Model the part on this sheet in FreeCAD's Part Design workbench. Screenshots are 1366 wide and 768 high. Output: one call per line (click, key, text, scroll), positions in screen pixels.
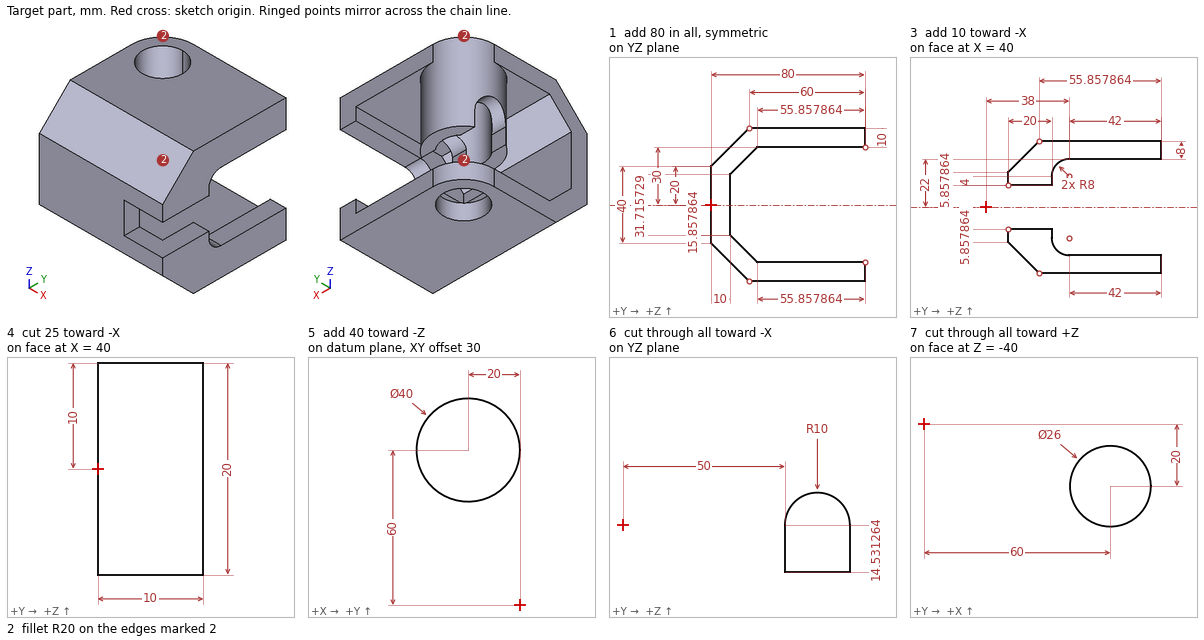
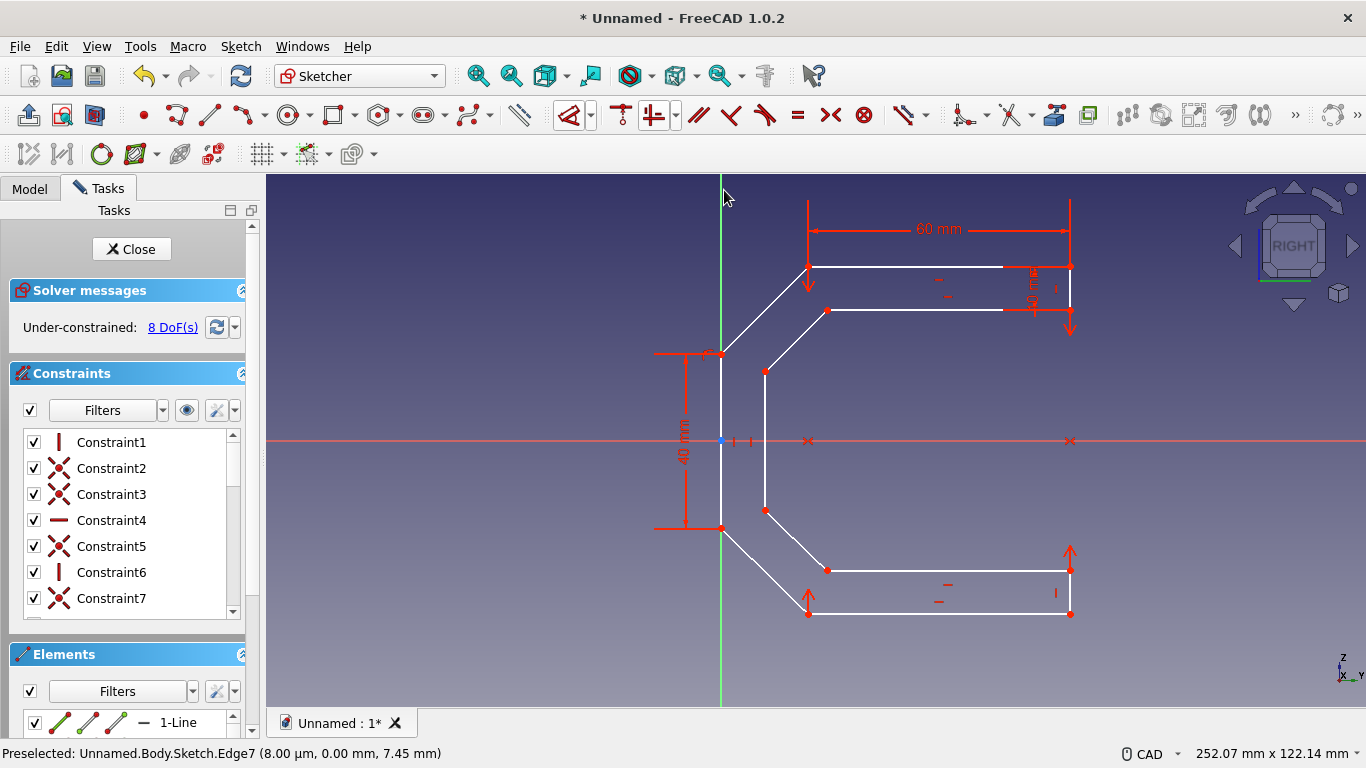
click(765, 511)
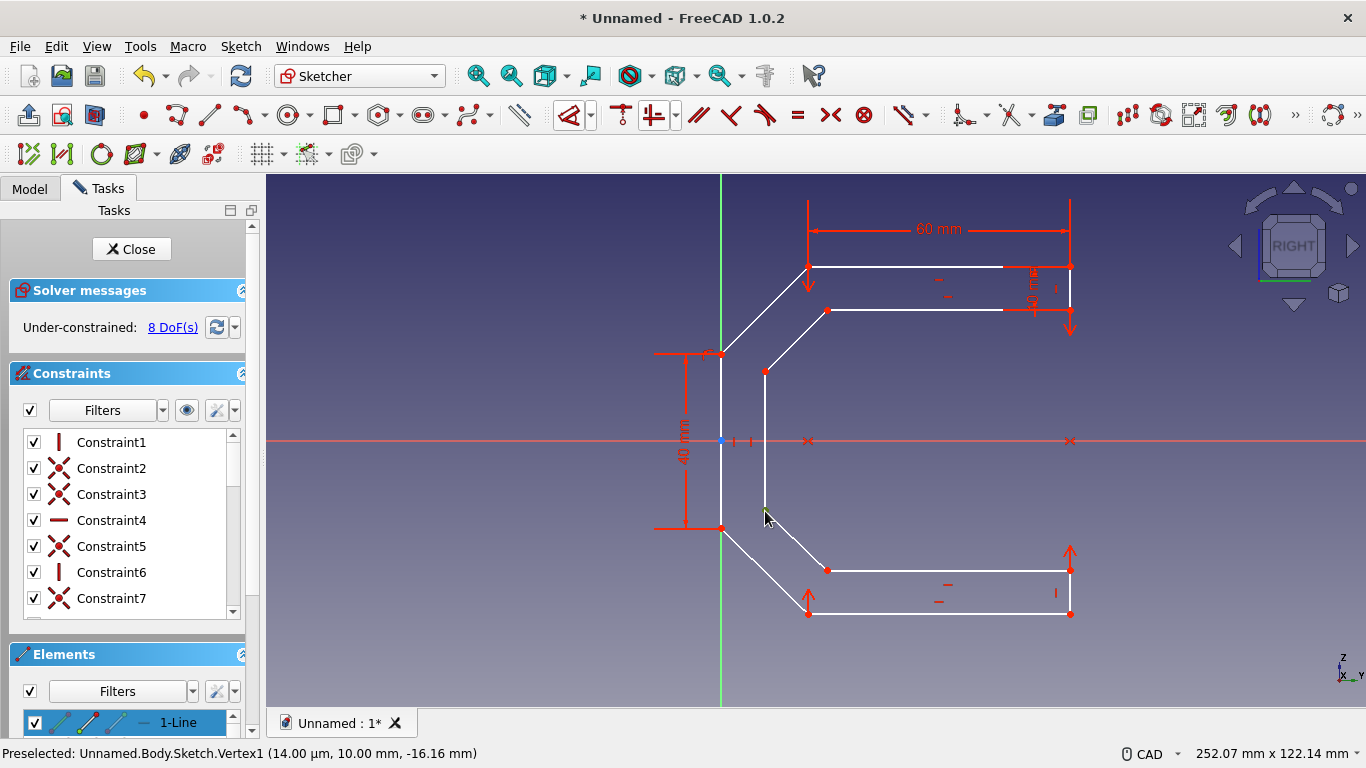
click(590, 116)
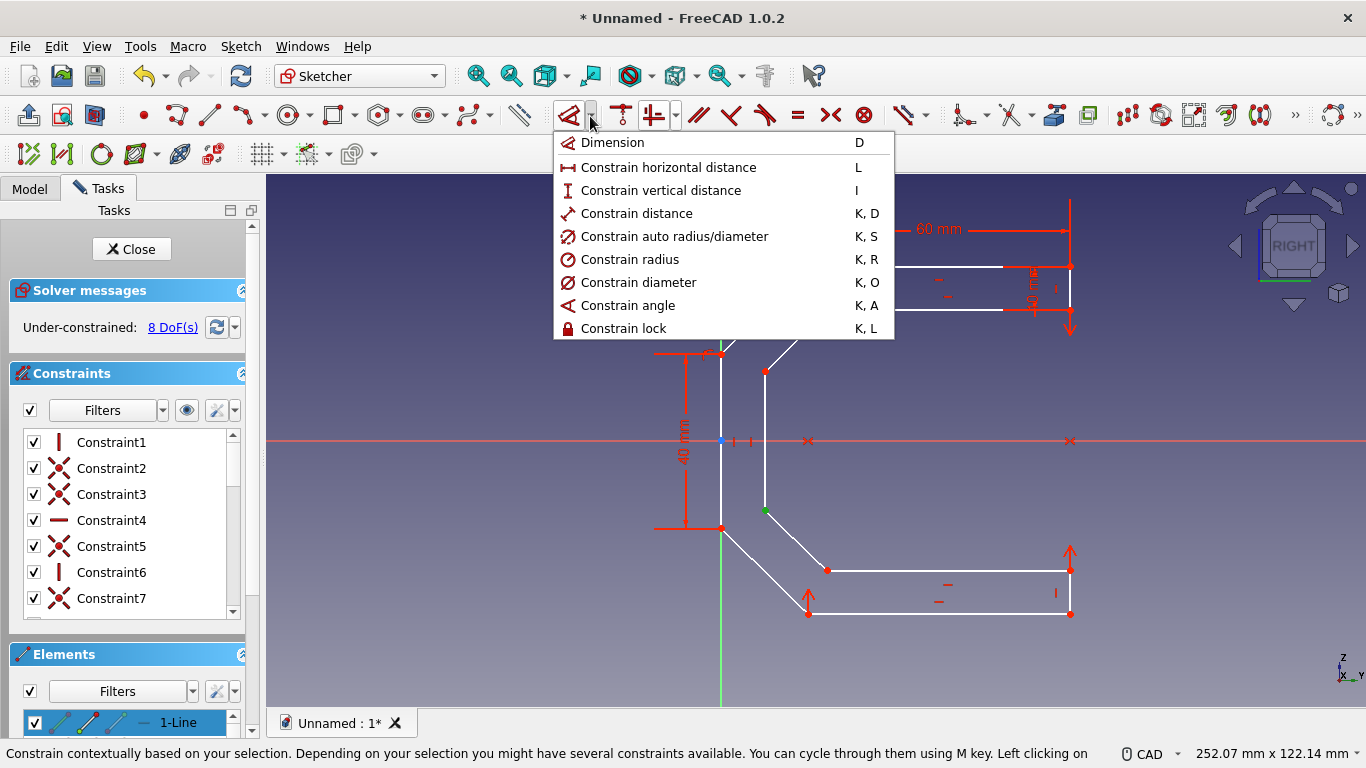
click(724, 168)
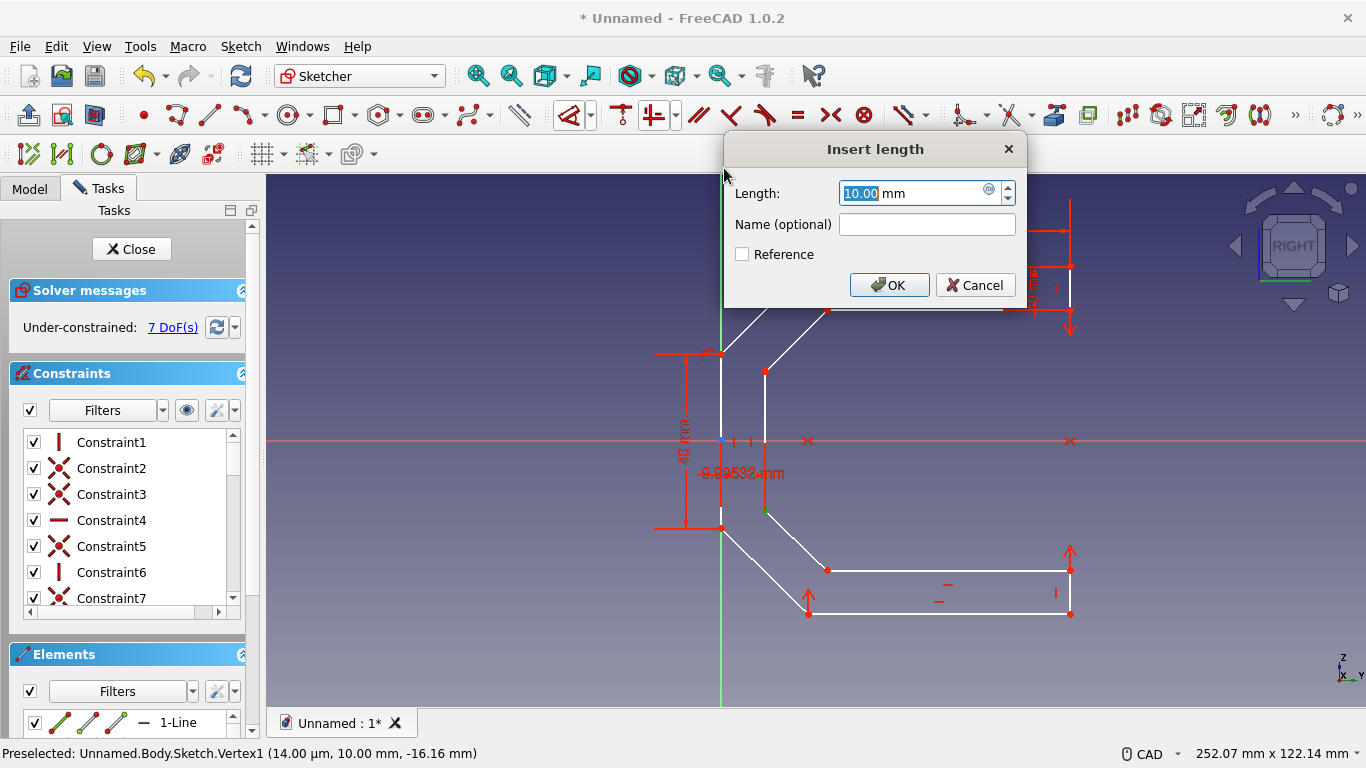
text(10)
key(Return)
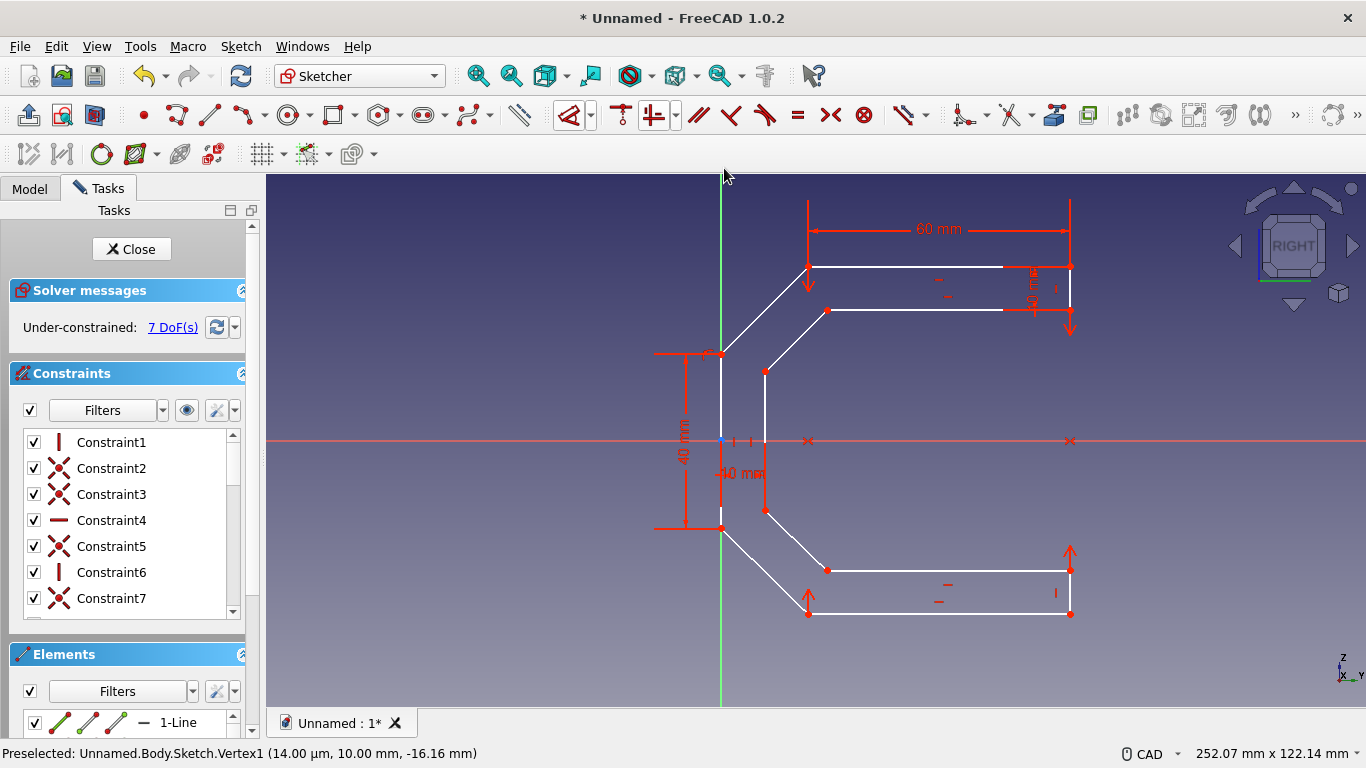
click(827, 310)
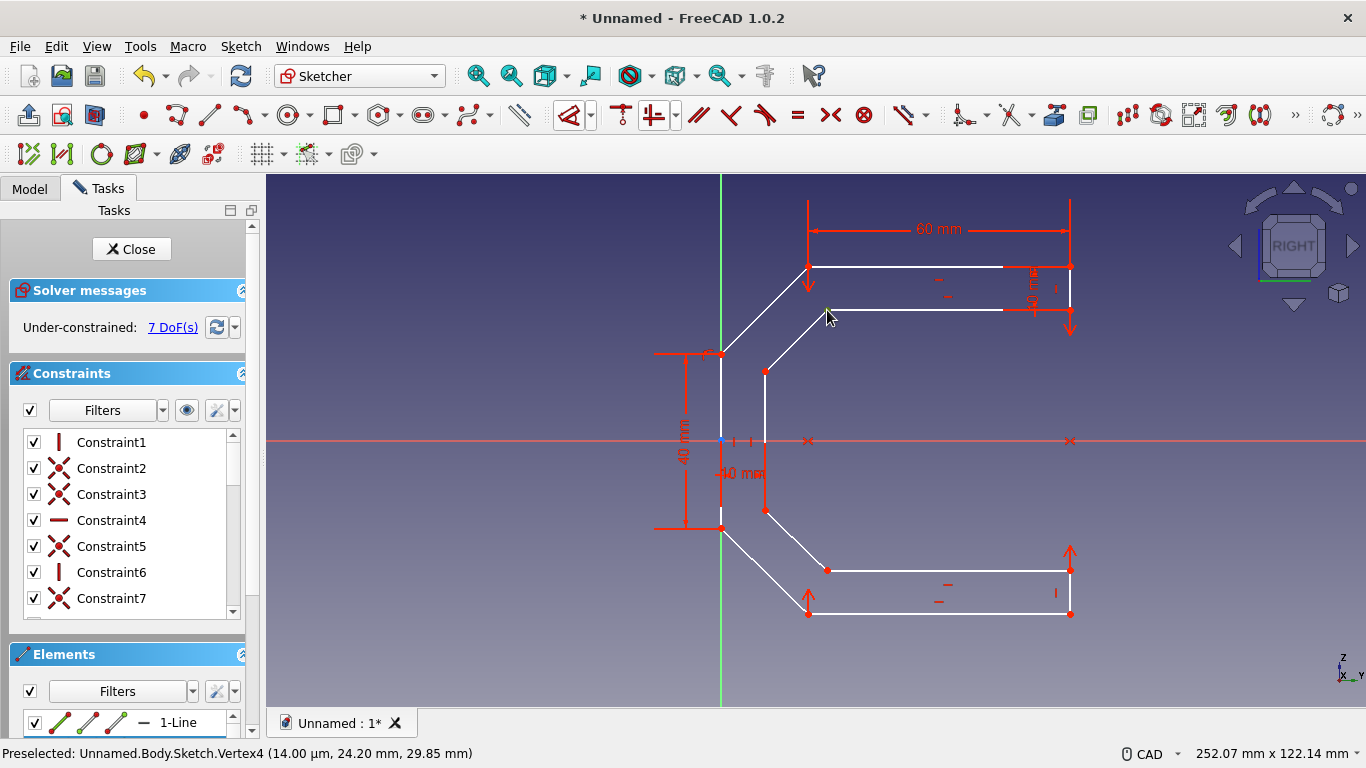
click(590, 116)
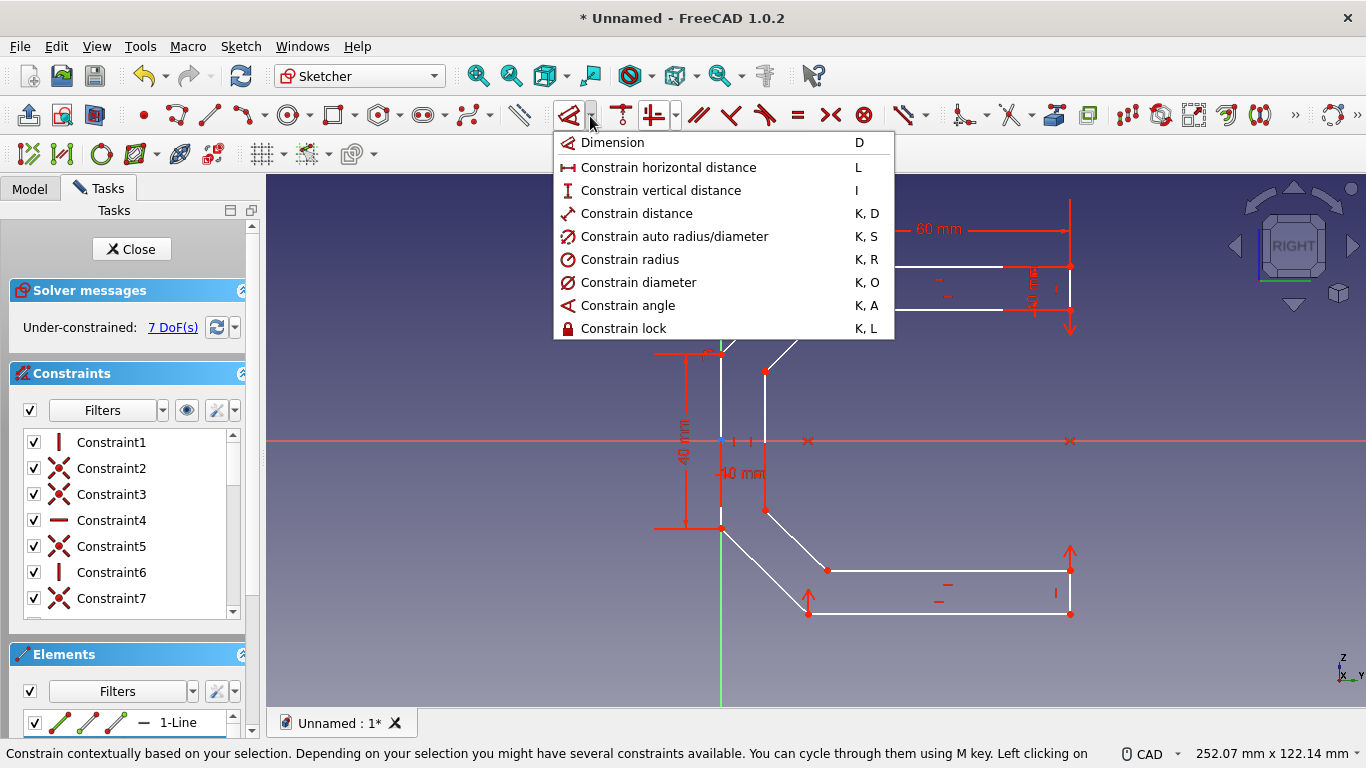
click(724, 190)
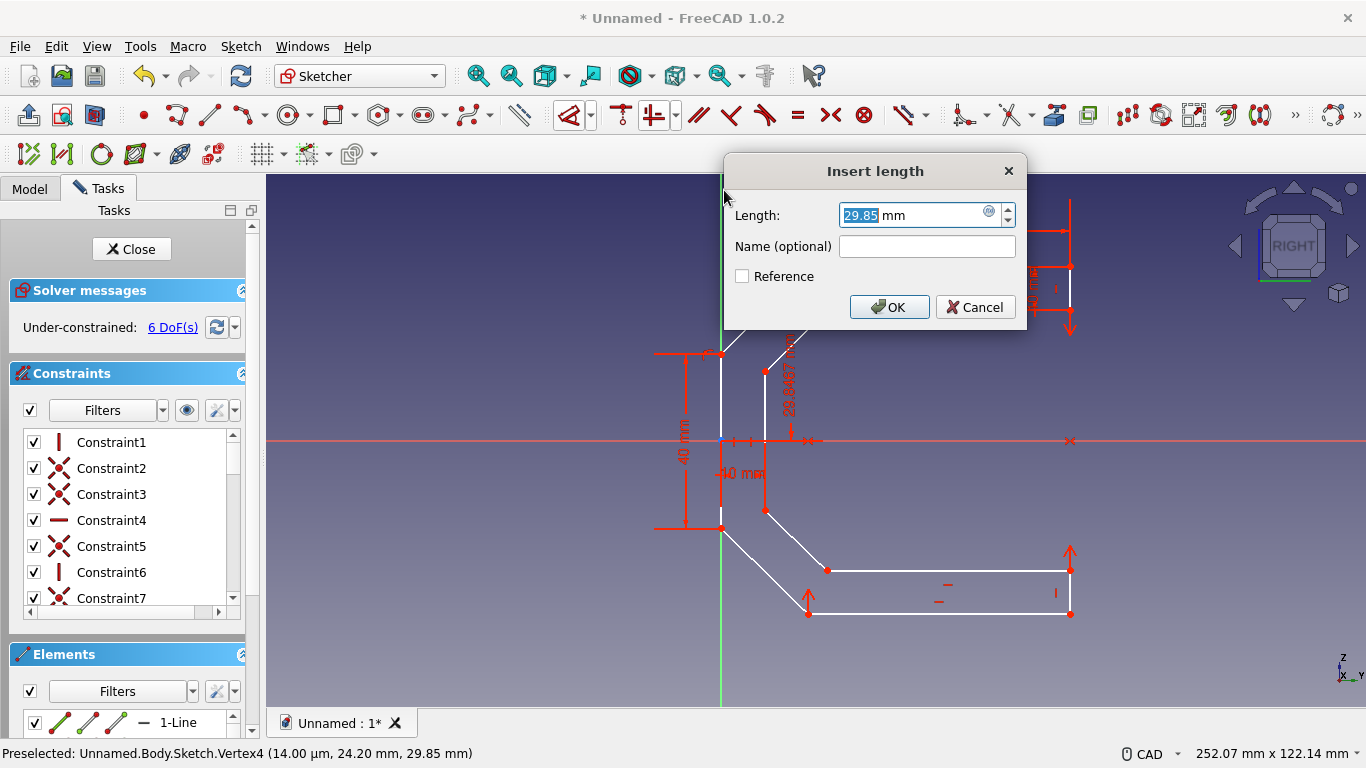
text(30)
key(Return)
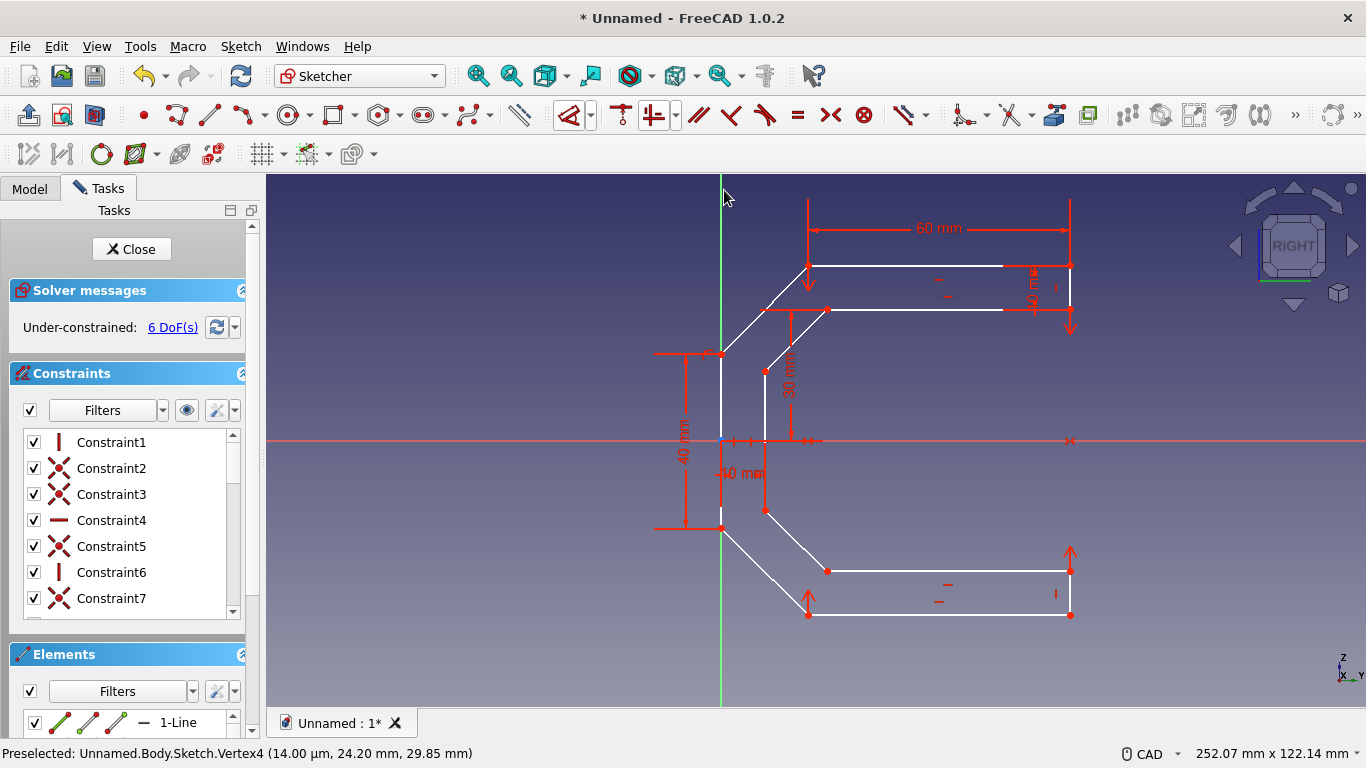
click(1070, 310)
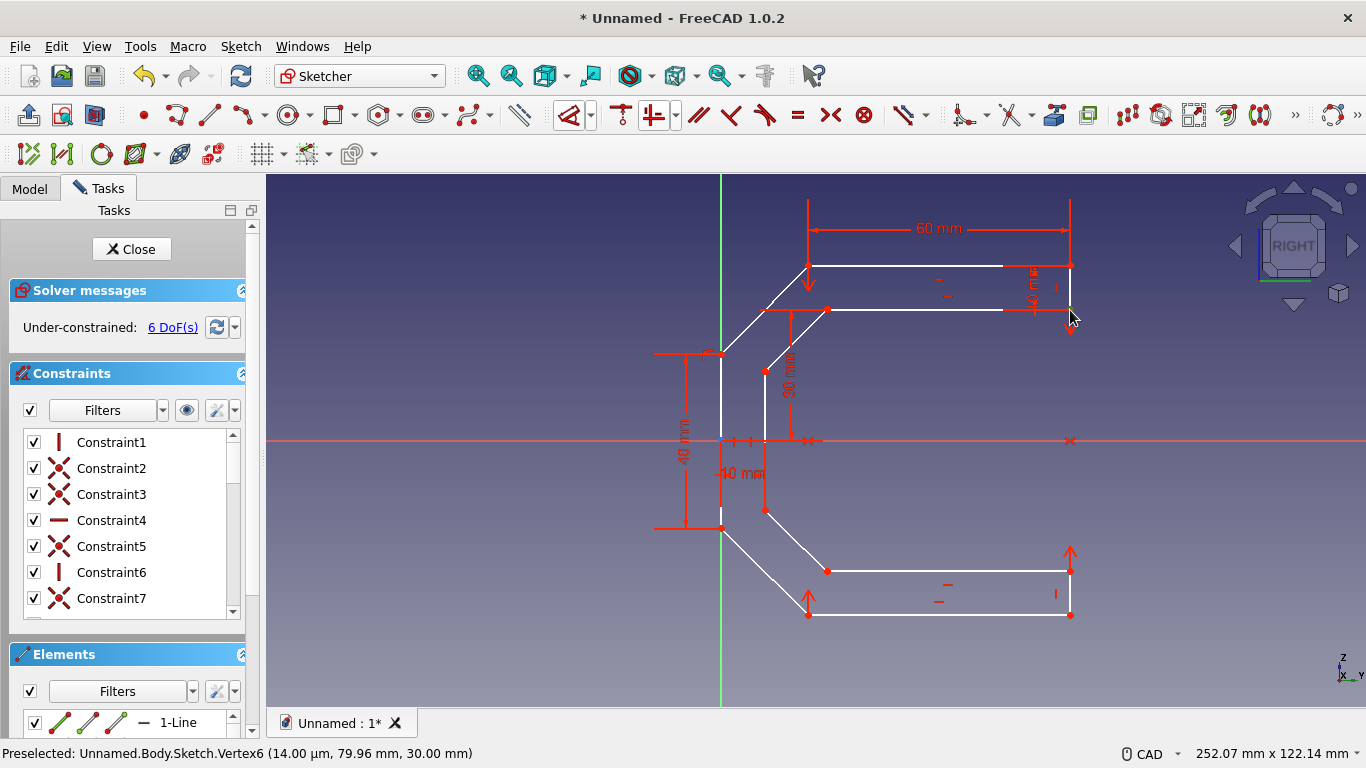
key(l)